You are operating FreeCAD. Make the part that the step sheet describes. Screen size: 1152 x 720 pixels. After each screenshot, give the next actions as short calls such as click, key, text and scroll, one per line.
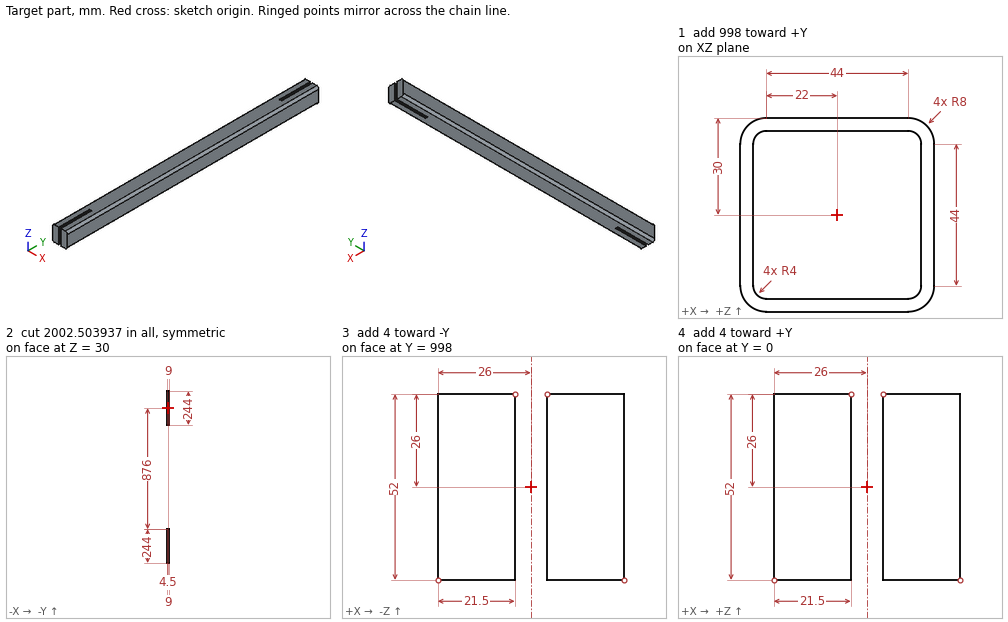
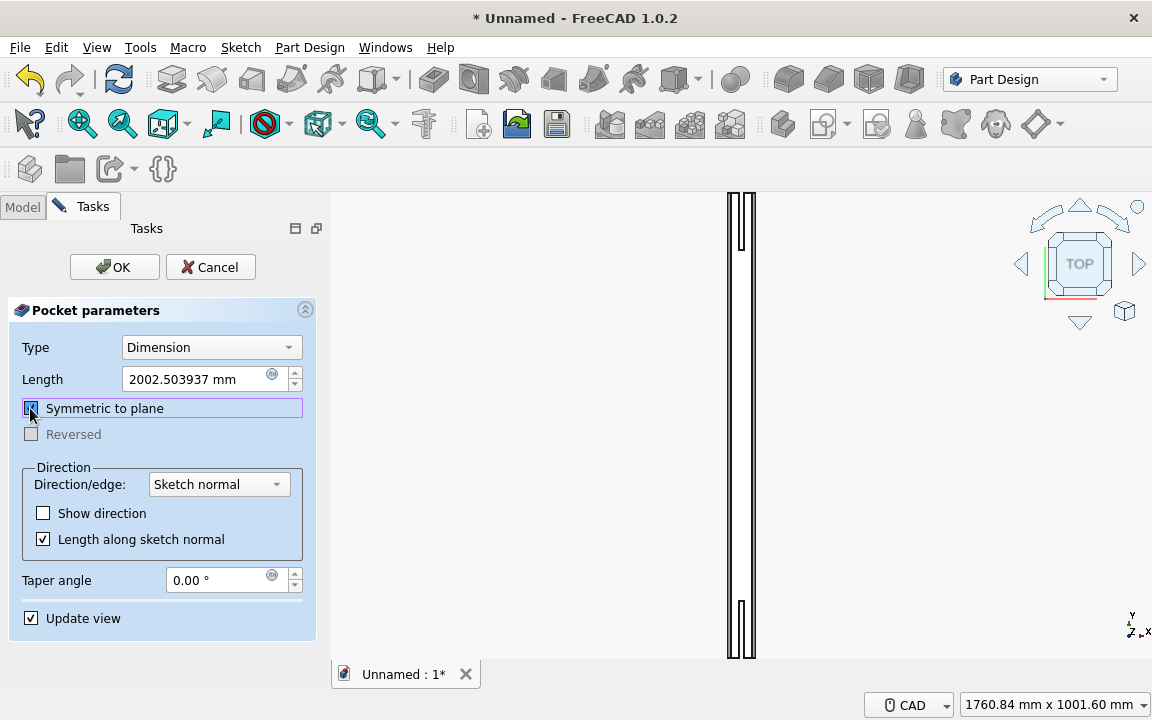
click(115, 267)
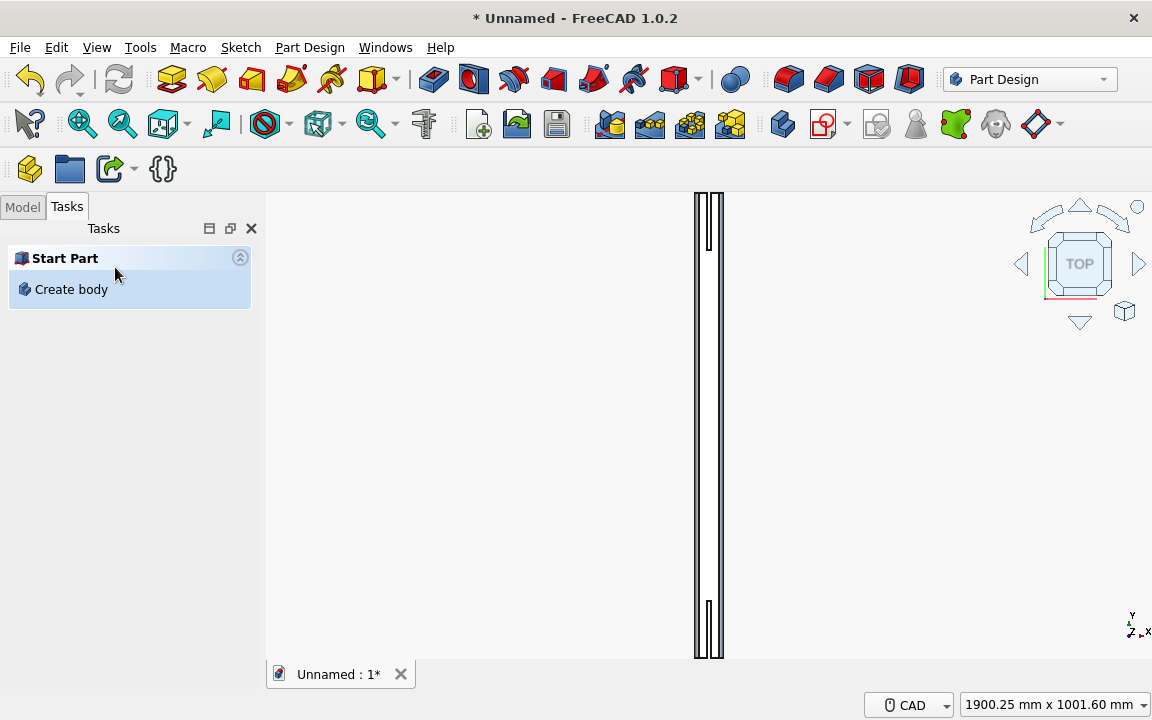
key(4)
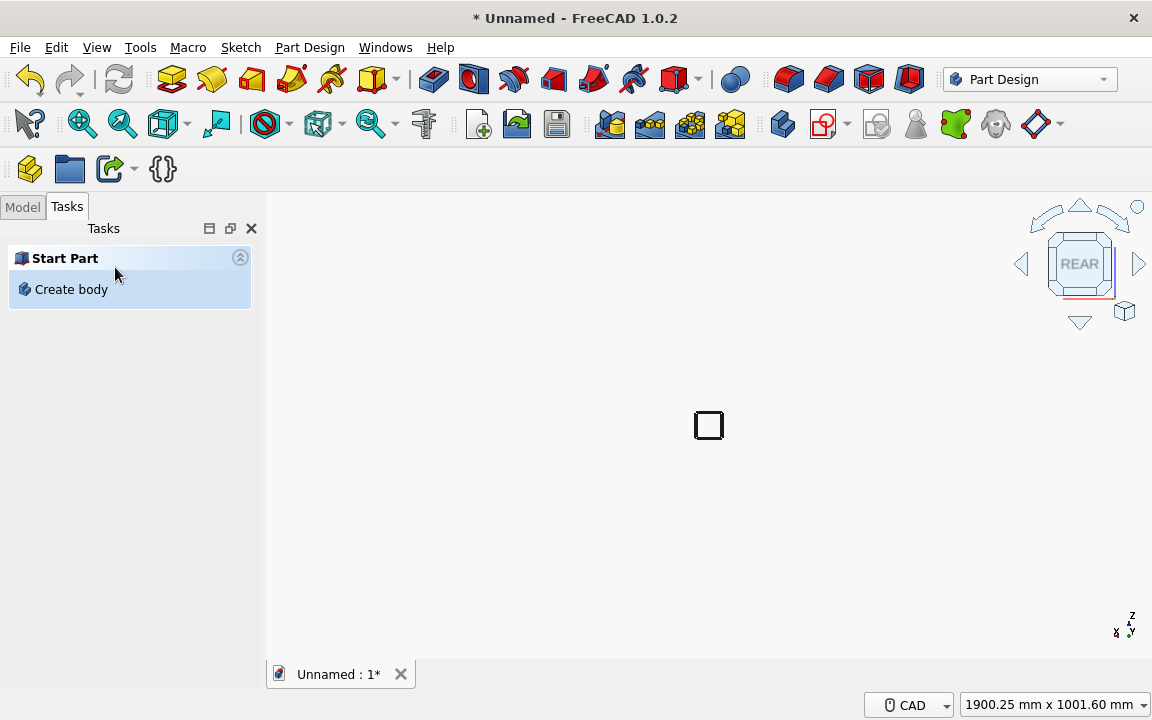
key(v)
key(f)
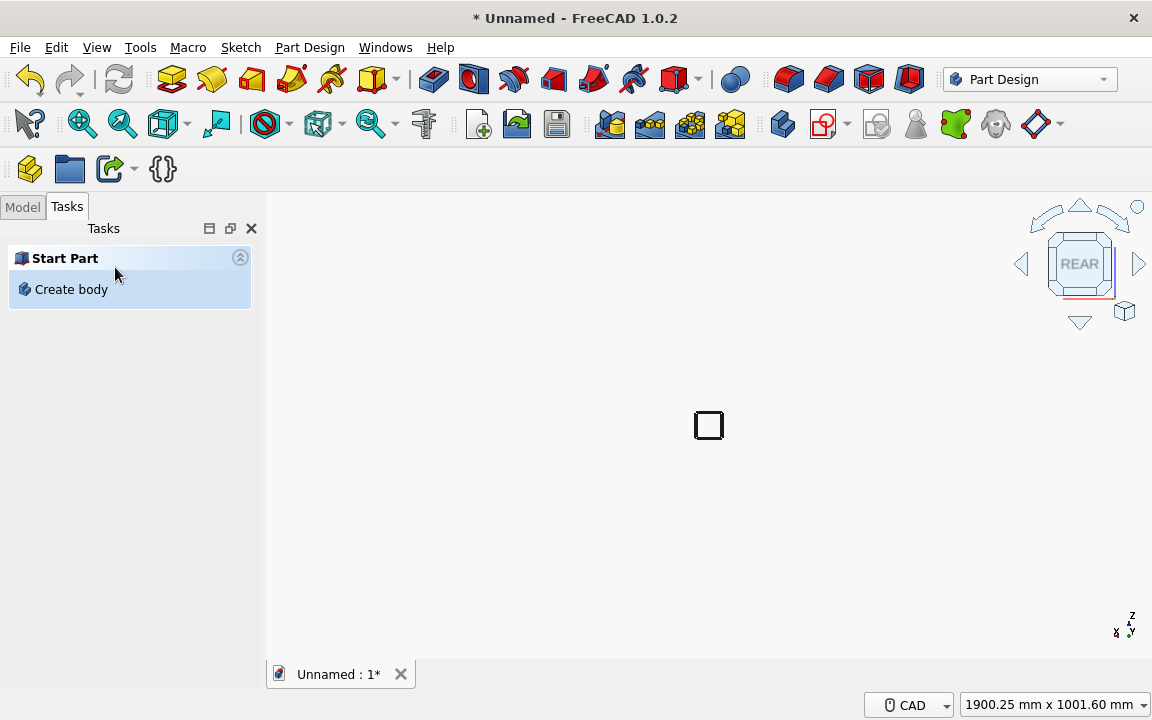
scroll(722, 417, up, 14)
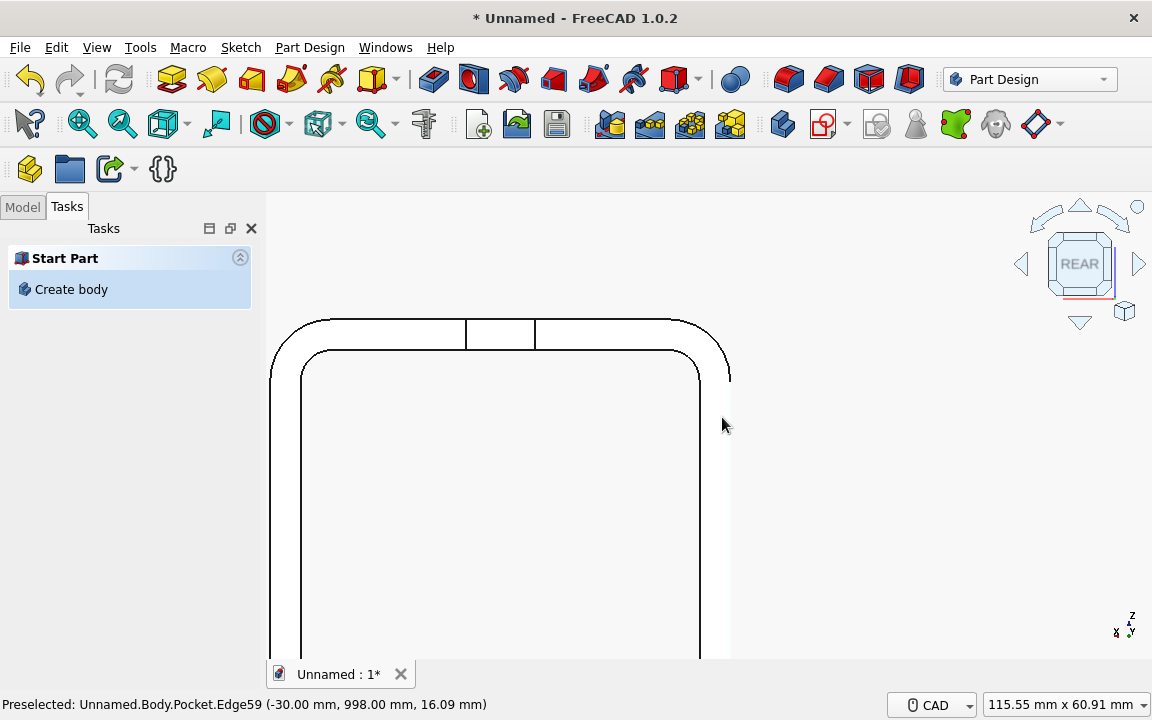
click(716, 417)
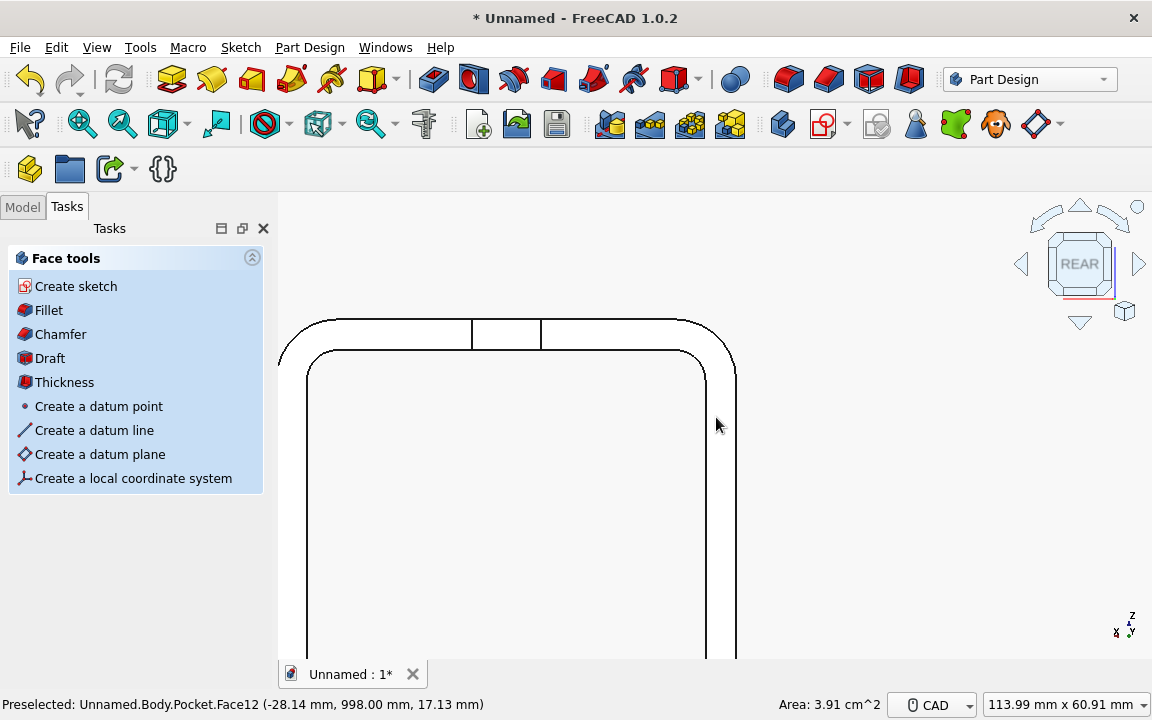
click(824, 124)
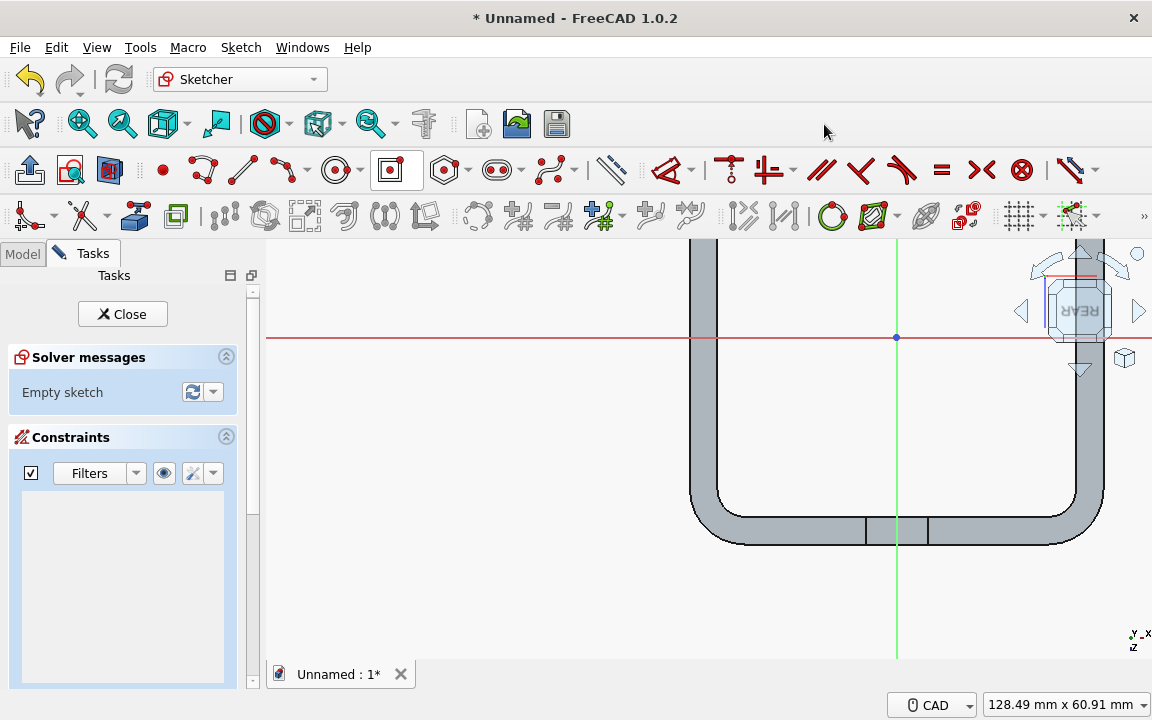
scroll(294, 631, down, 2)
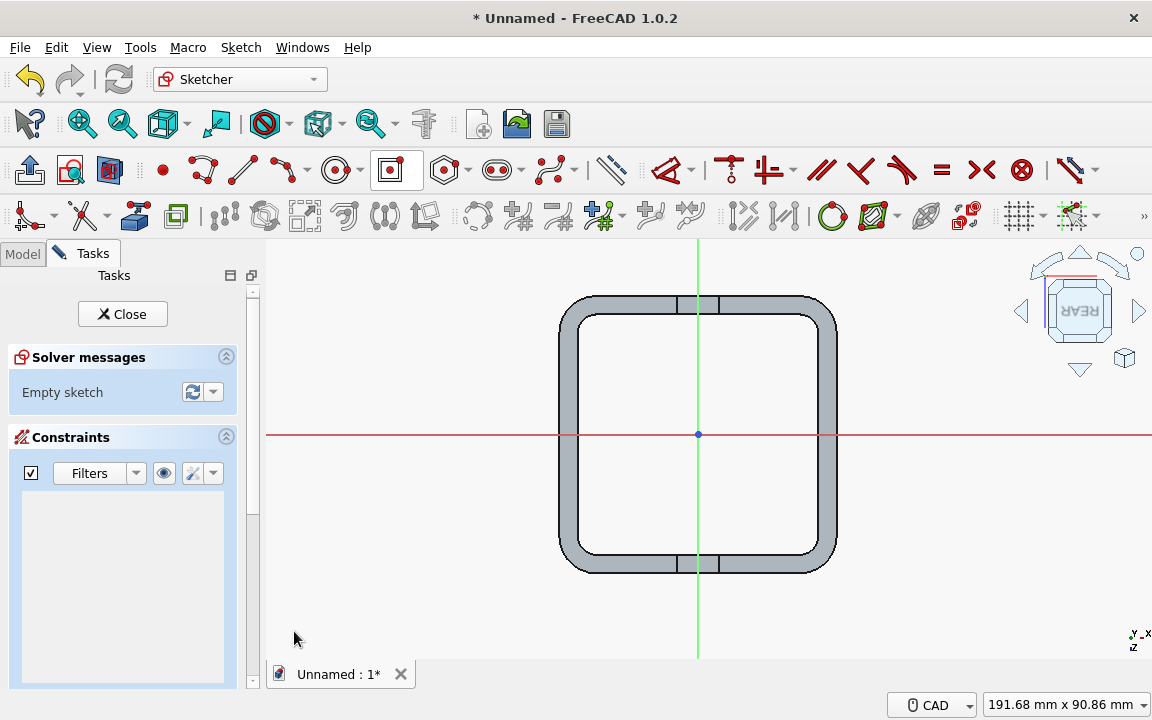
click(418, 170)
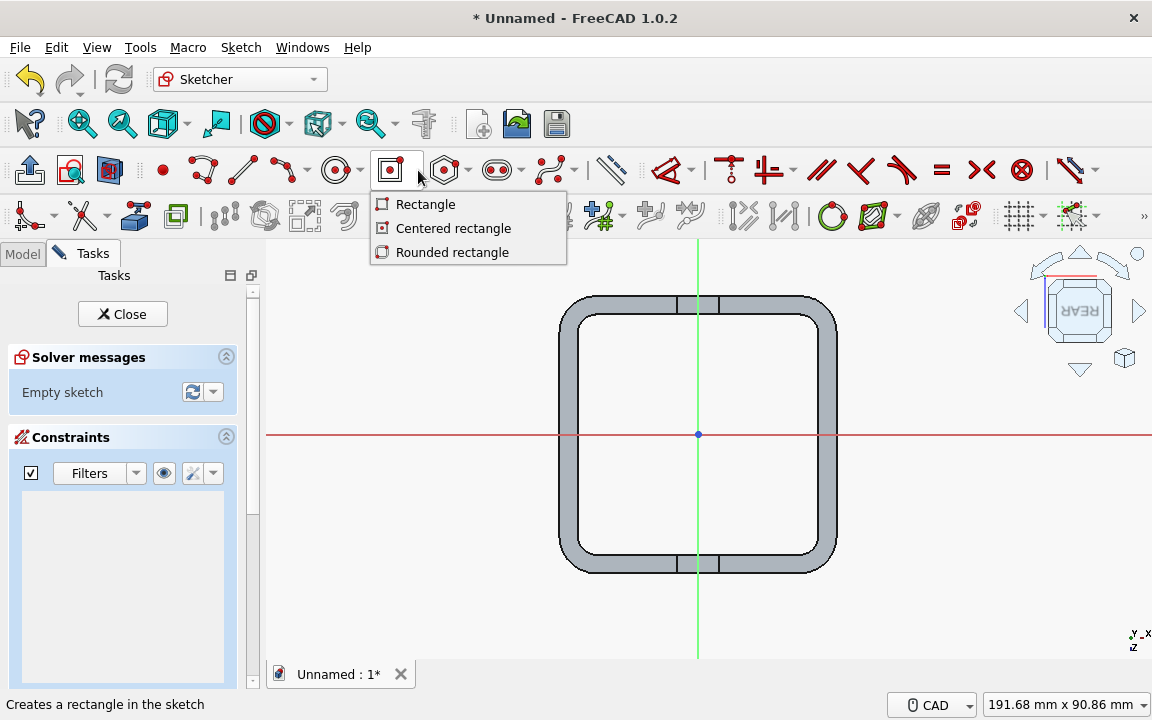
click(468, 204)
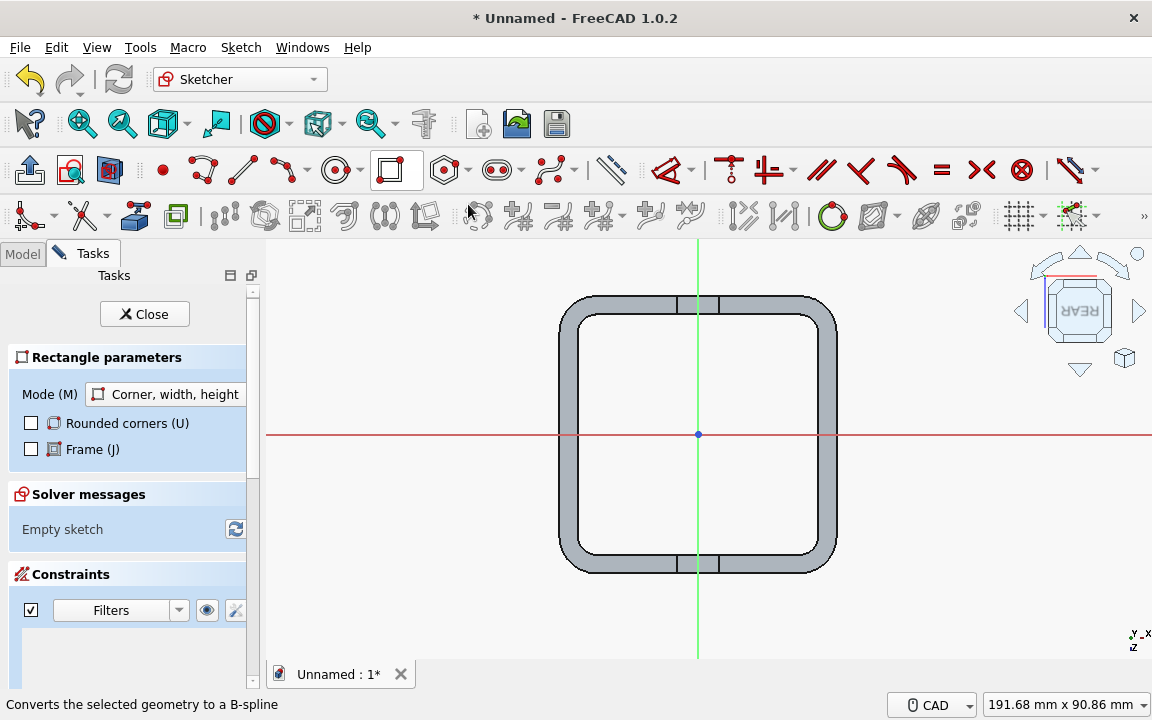
click(578, 314)
click(677, 555)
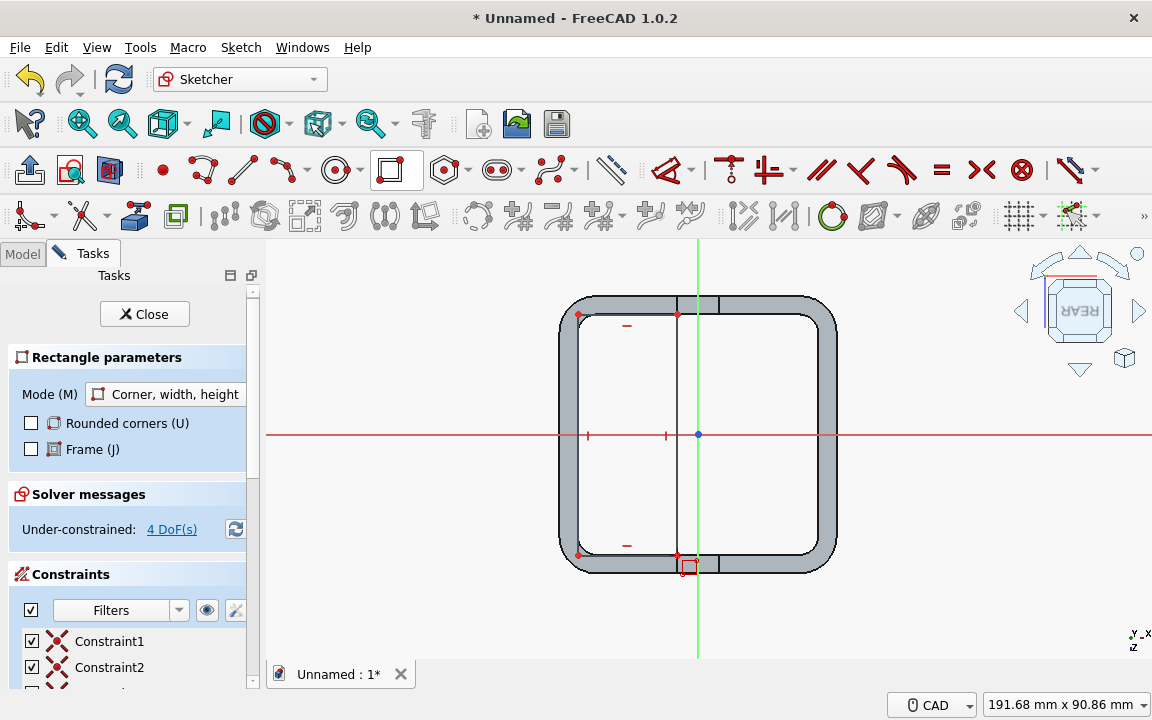
click(719, 314)
click(818, 555)
key(Escape)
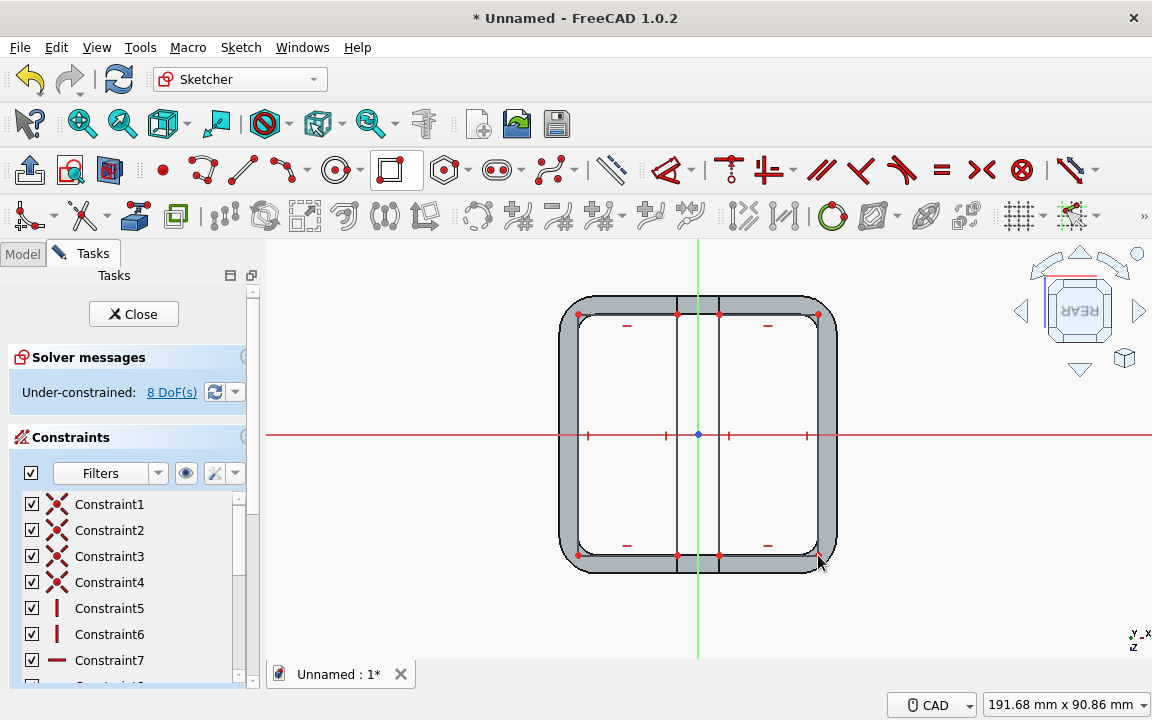
click(677, 315)